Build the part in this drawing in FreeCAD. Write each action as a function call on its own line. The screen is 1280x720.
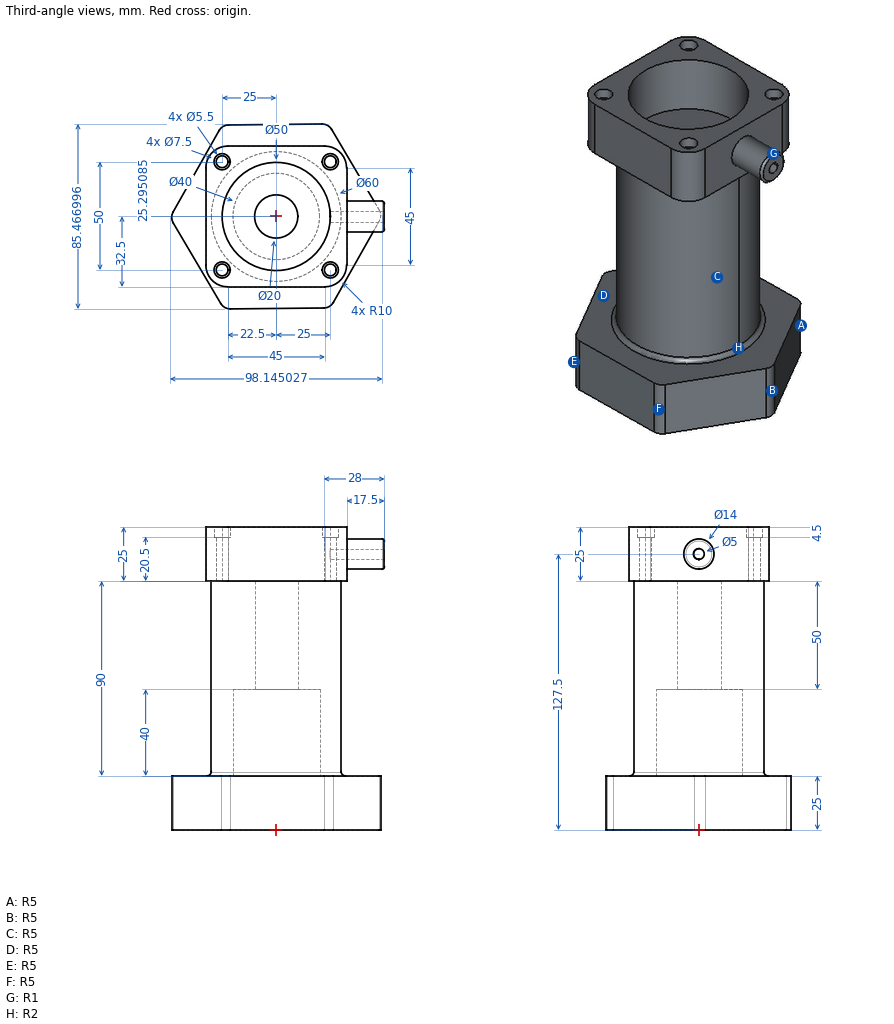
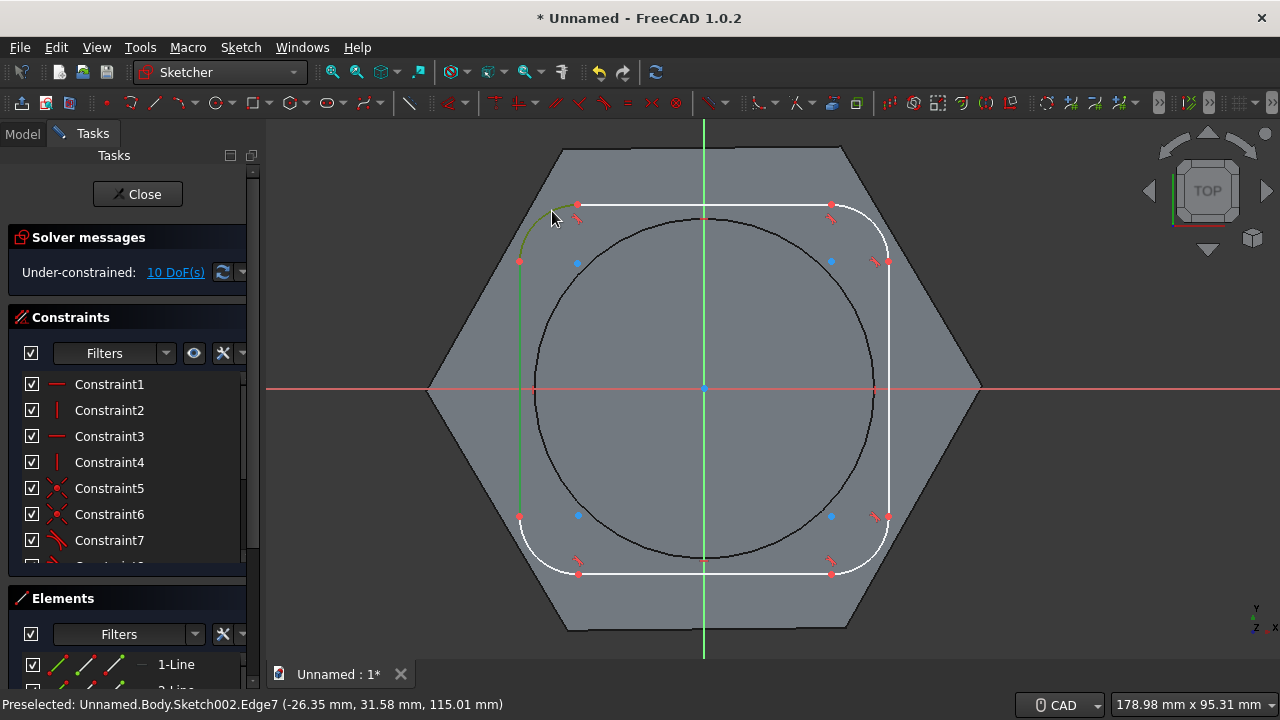
click(604, 104)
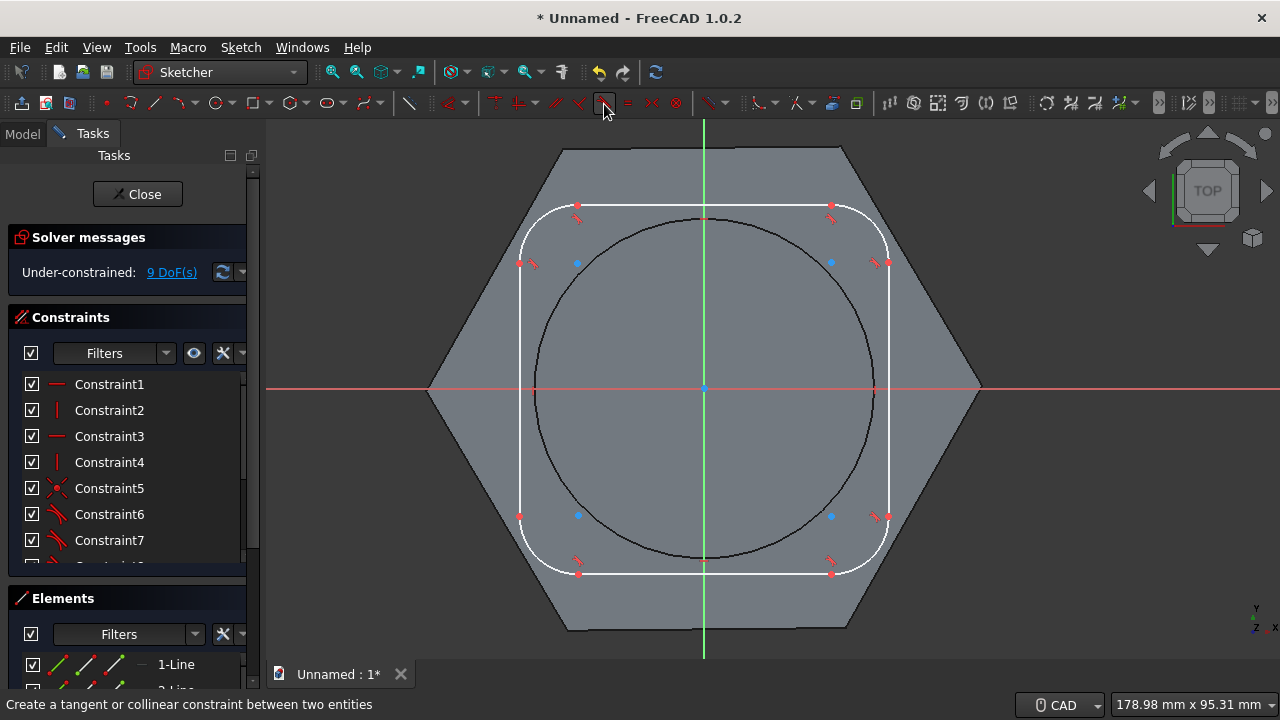
click(520, 339)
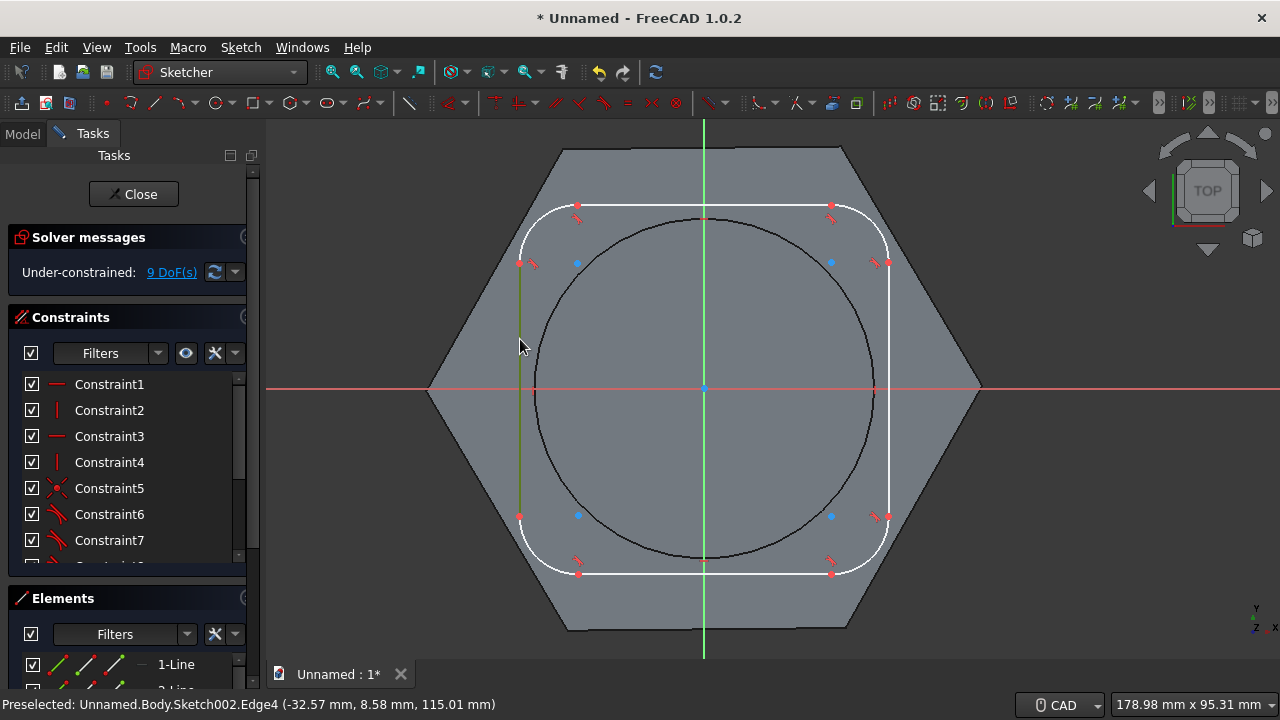
click(526, 543)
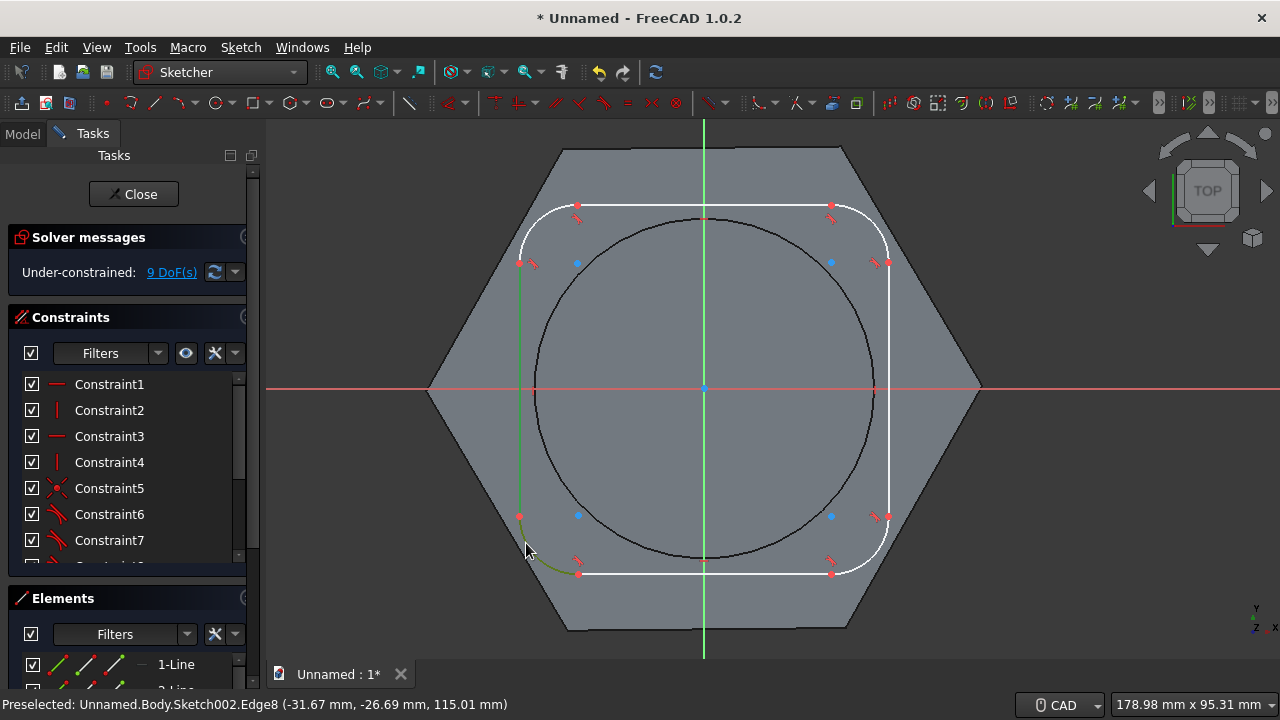
click(604, 104)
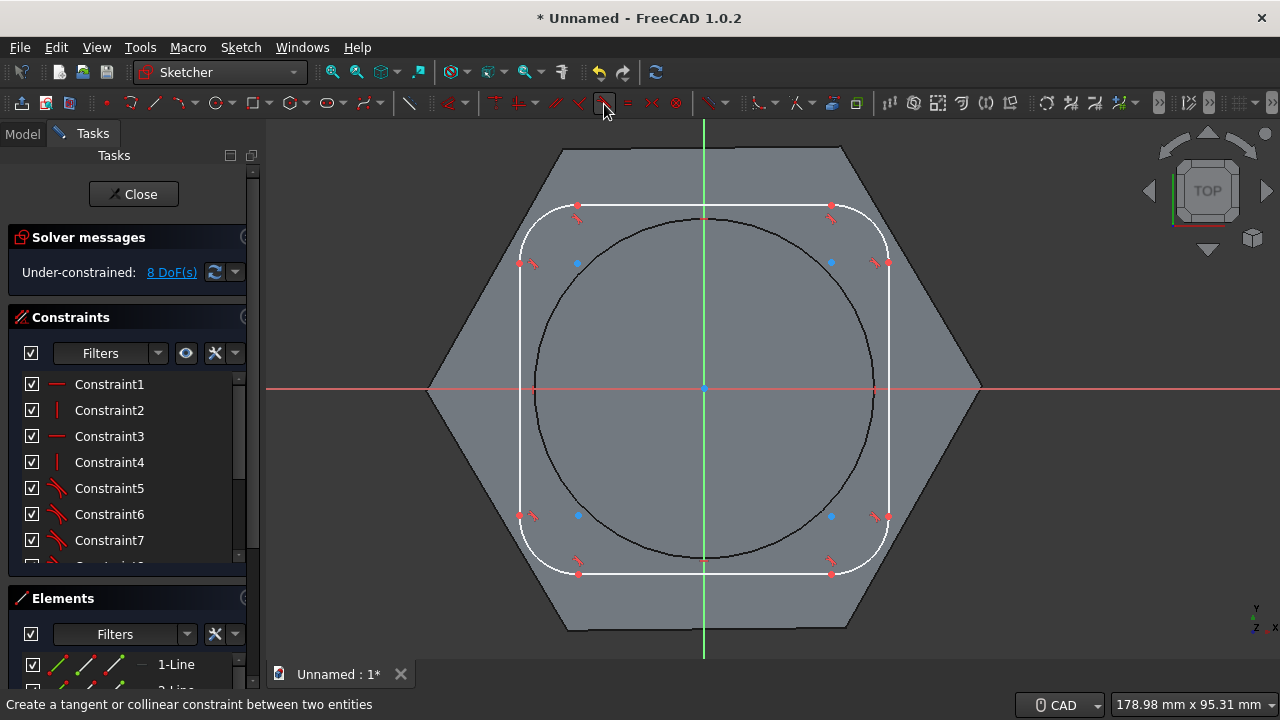
click(857, 568)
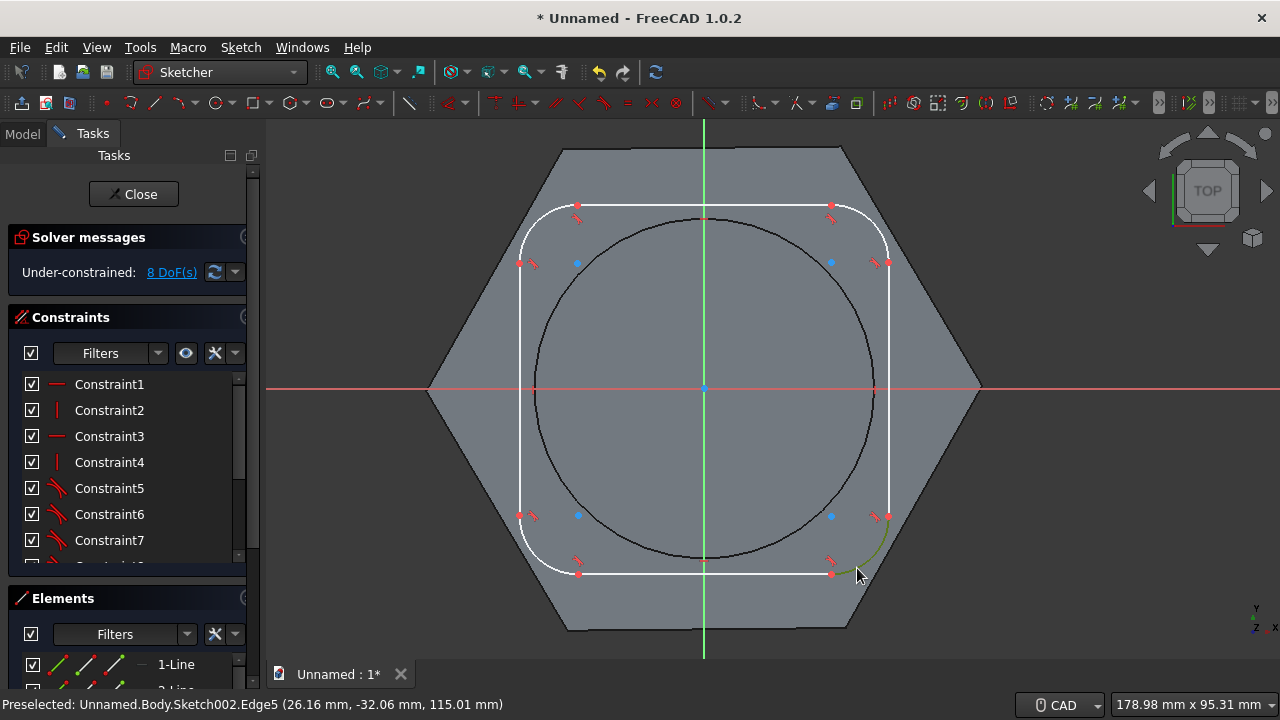
click(882, 236)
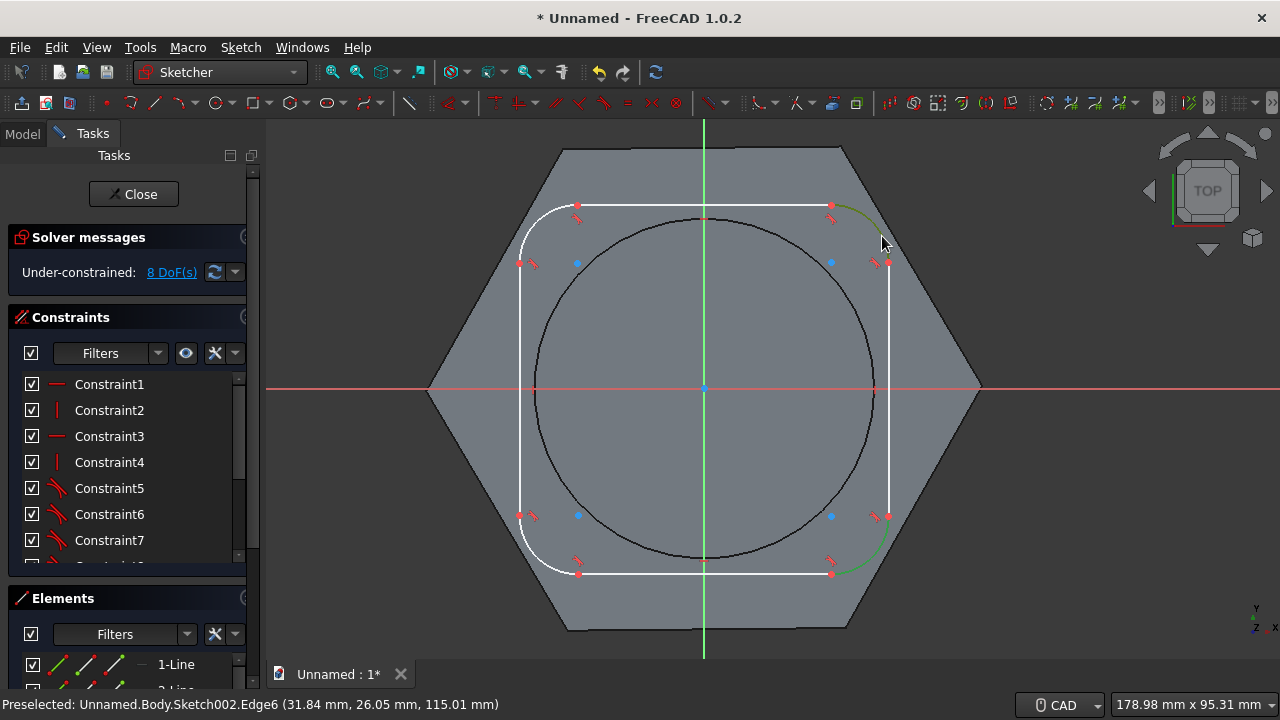
click(551, 211)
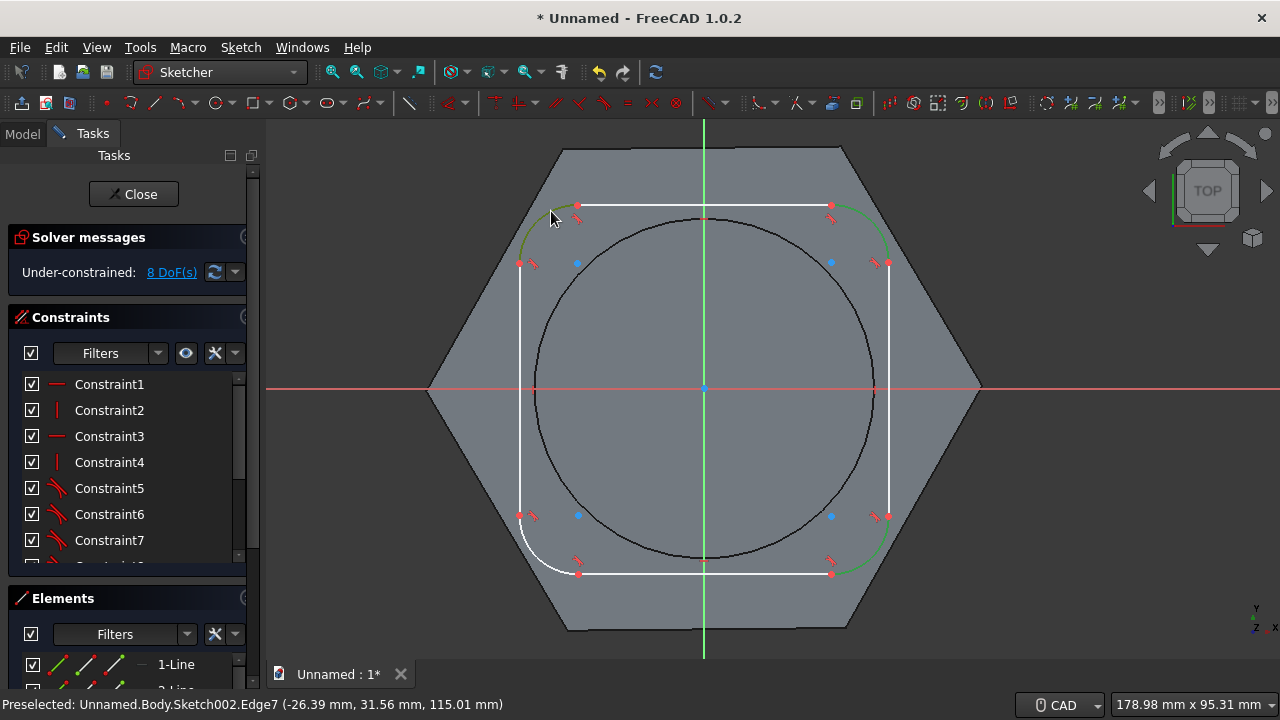
click(526, 542)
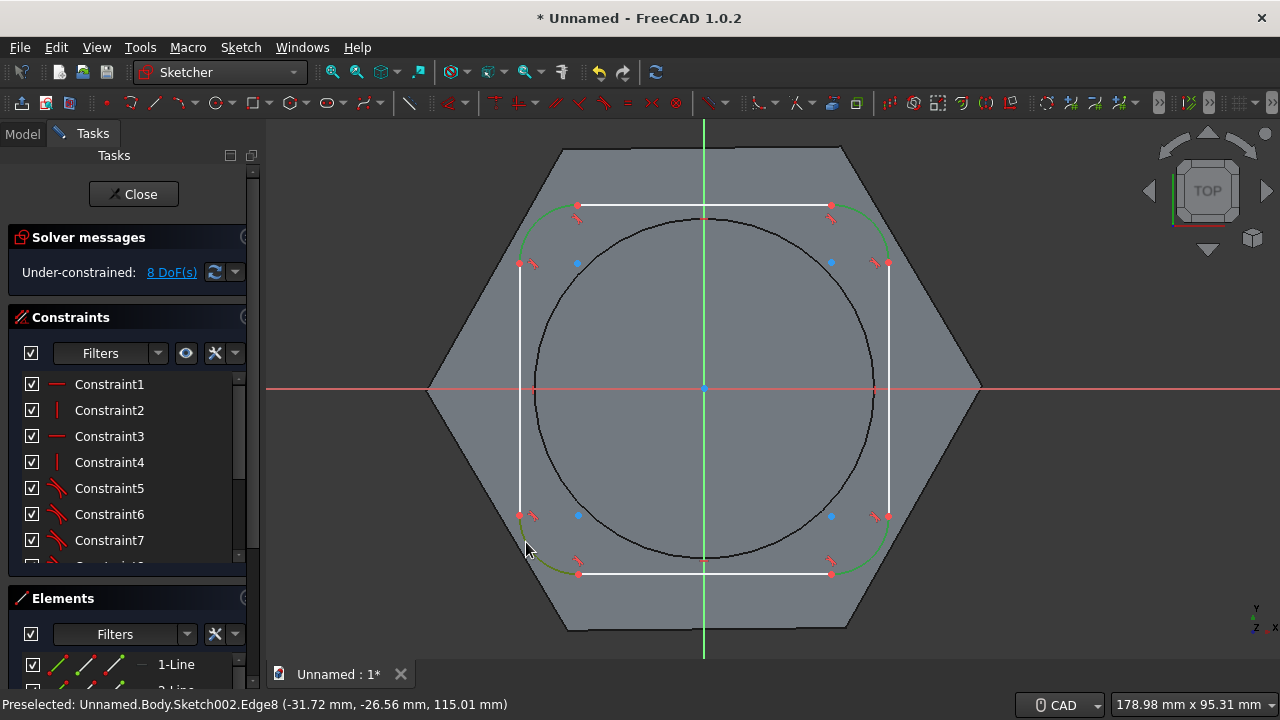
click(628, 104)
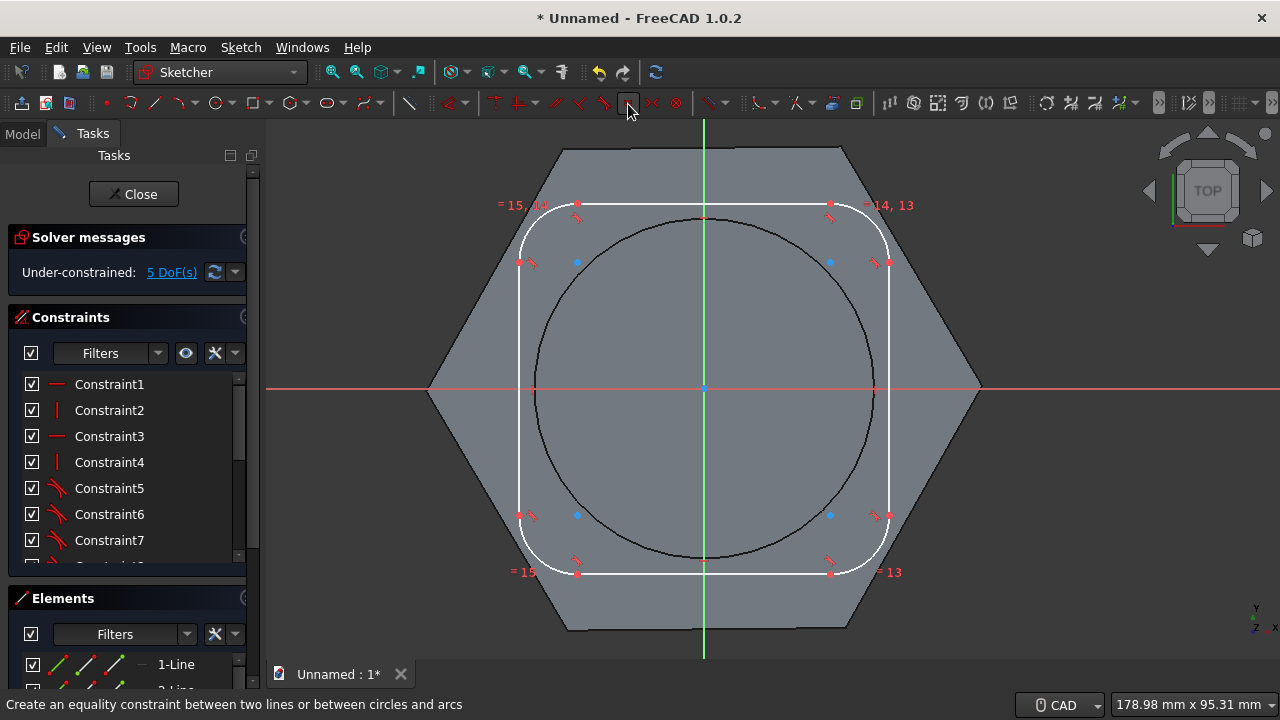
click(448, 104)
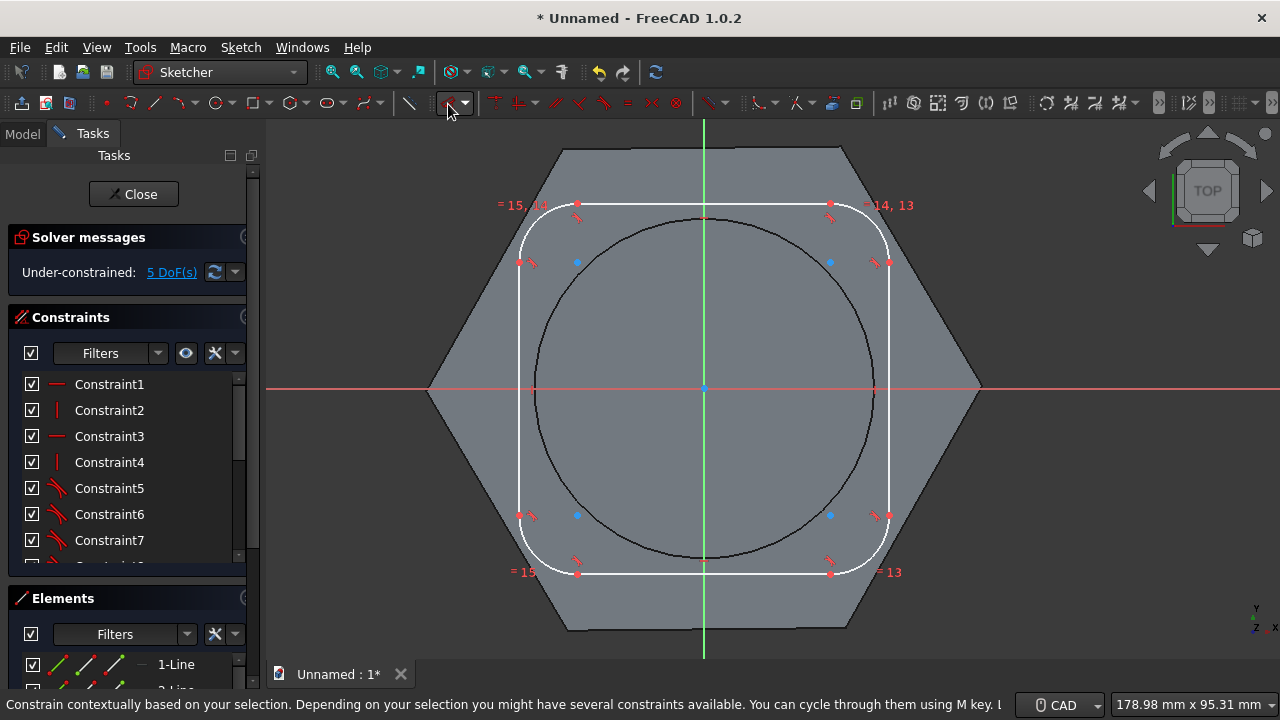
click(857, 568)
click(871, 597)